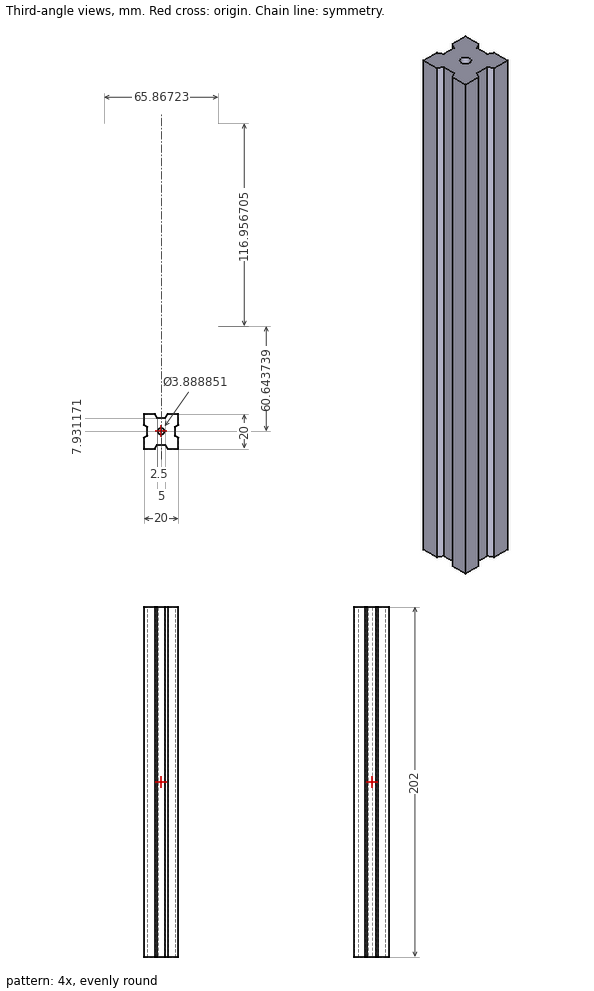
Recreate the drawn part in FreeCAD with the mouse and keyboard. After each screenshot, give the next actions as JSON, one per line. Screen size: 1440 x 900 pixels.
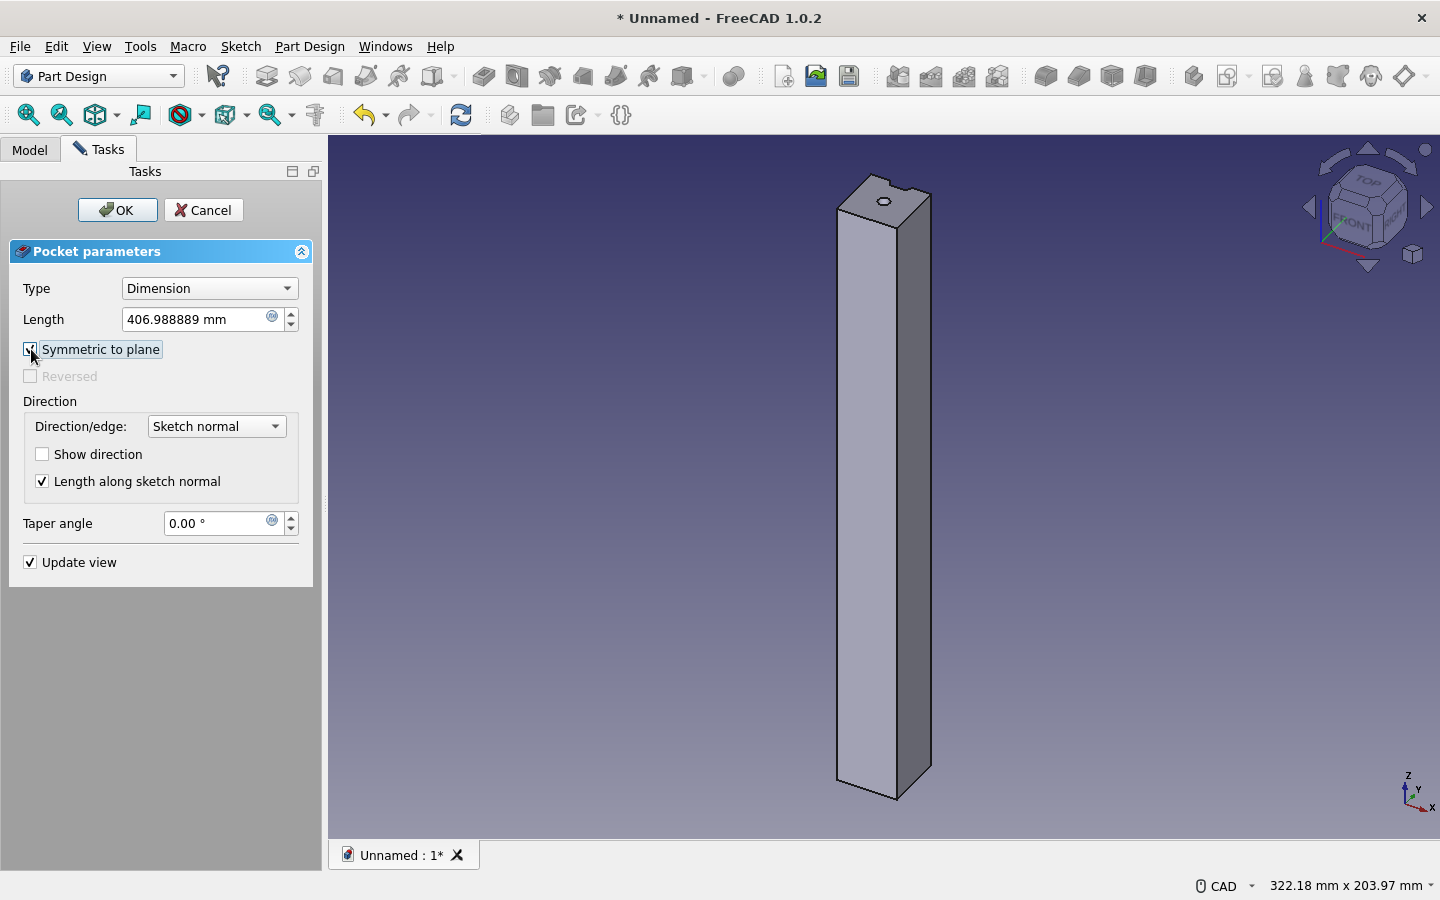
{"action": "left_click", "coordinate": [118, 210]}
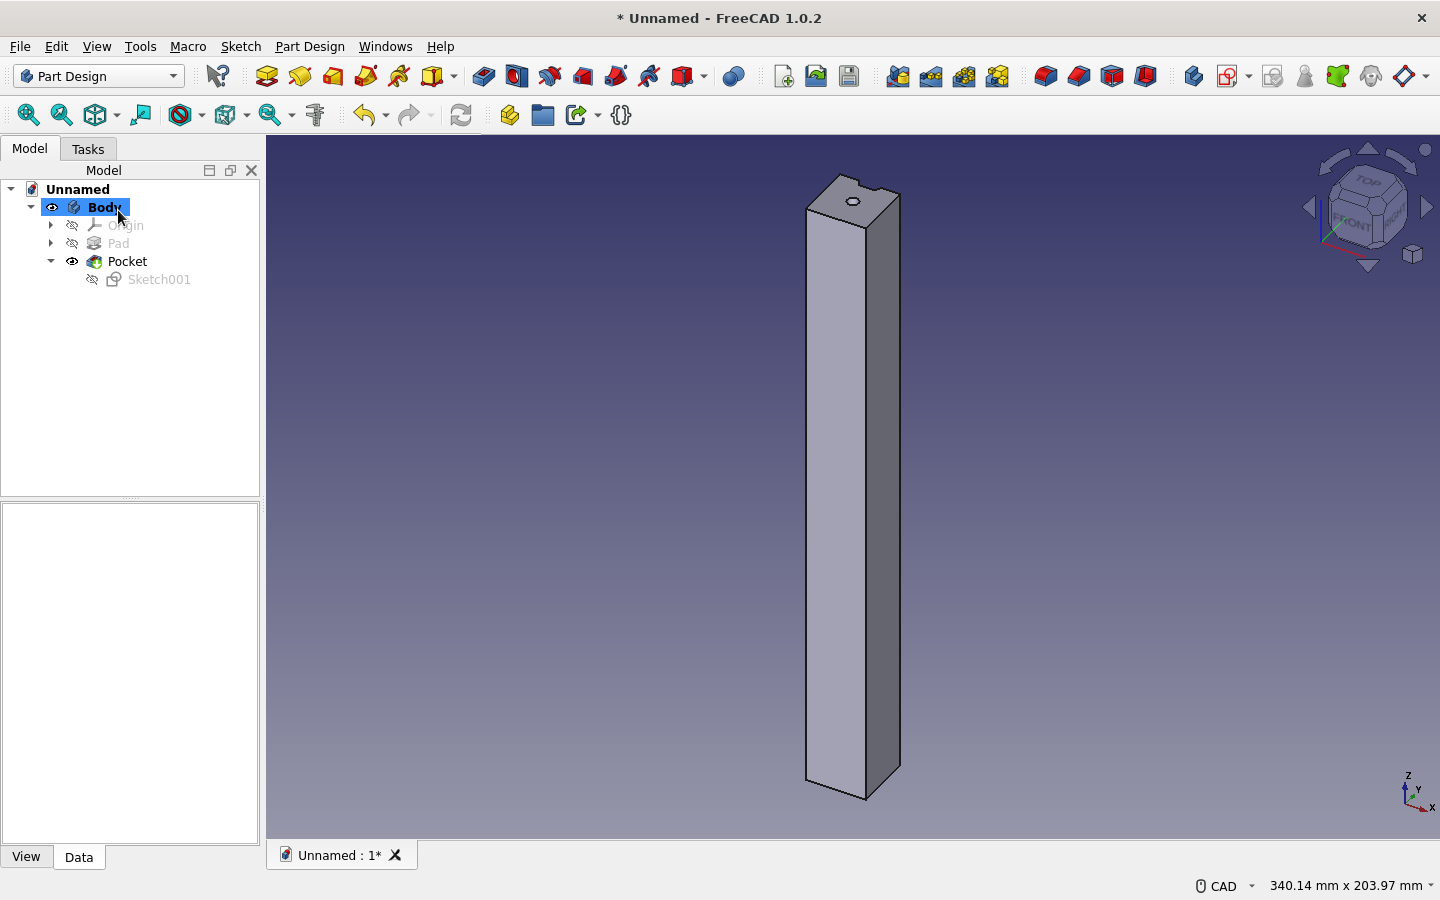
{"action": "left_click", "coordinate": [117, 261]}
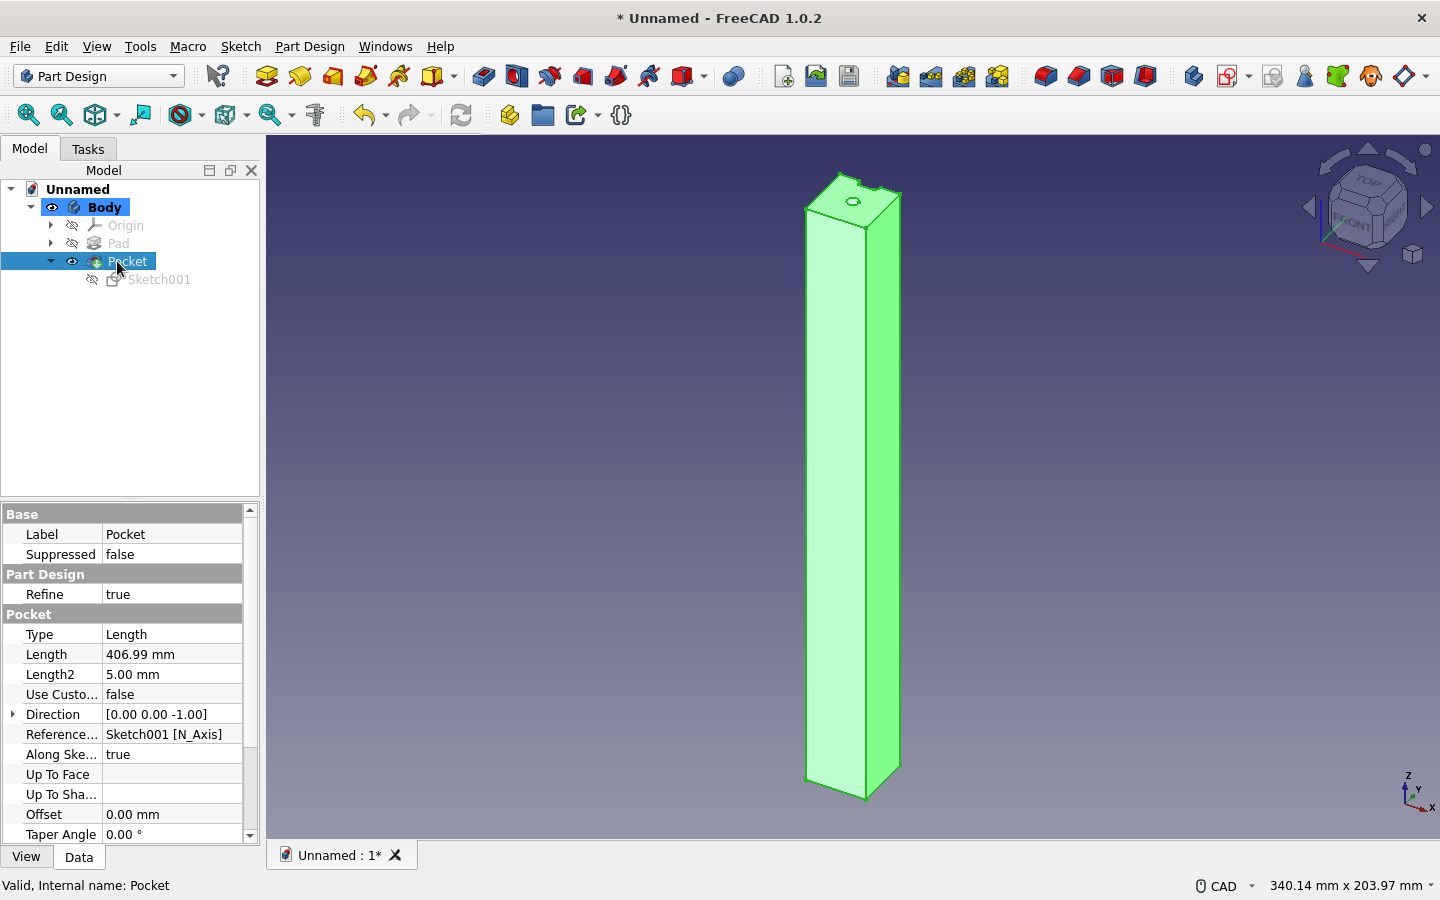
{"action": "left_click", "coordinate": [964, 76]}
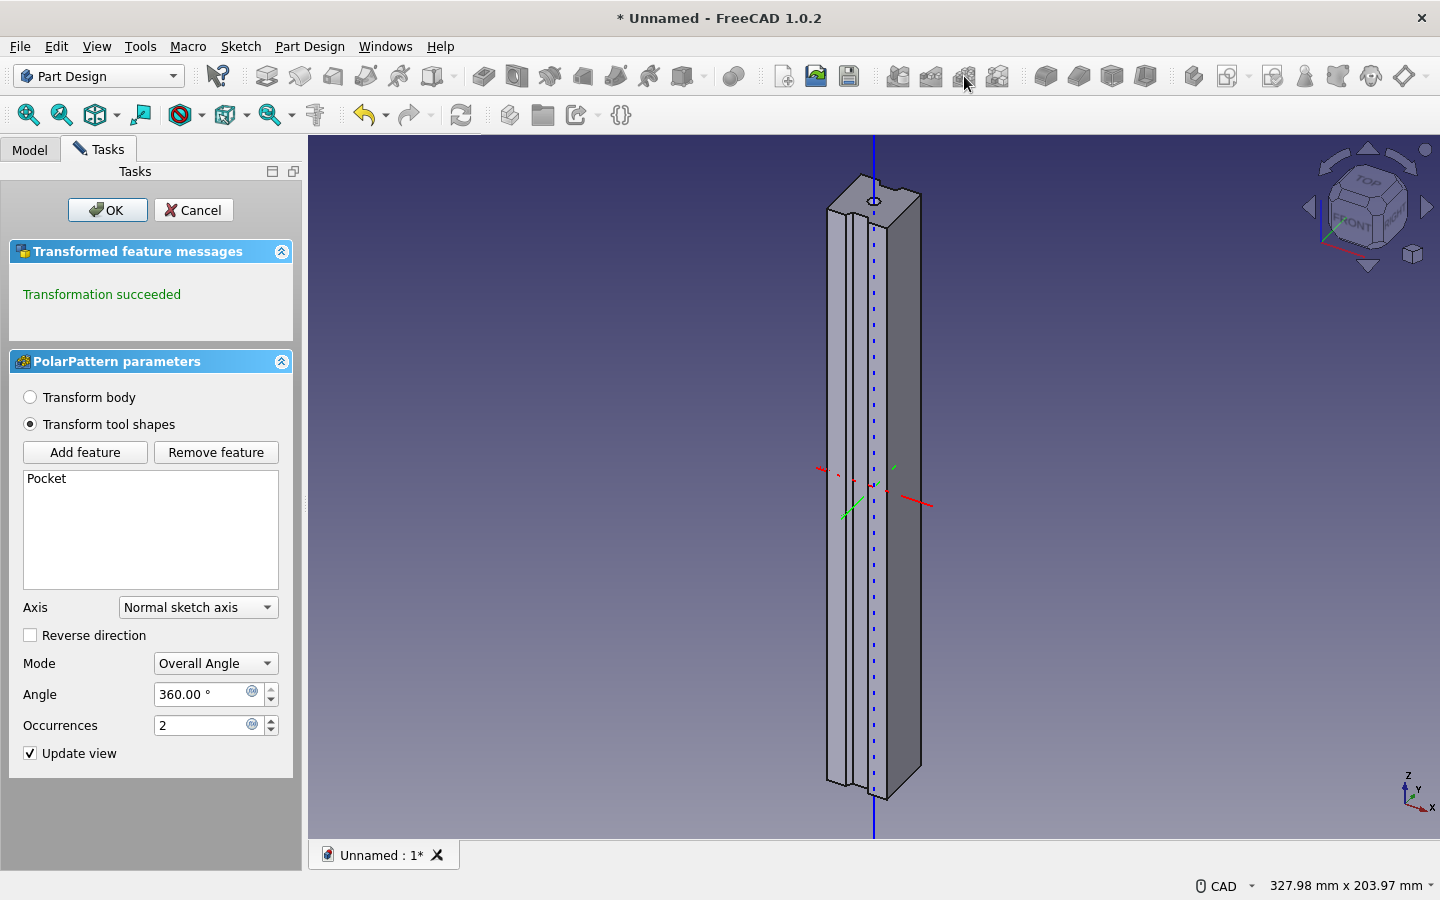
{"action": "left_click", "coordinate": [199, 608]}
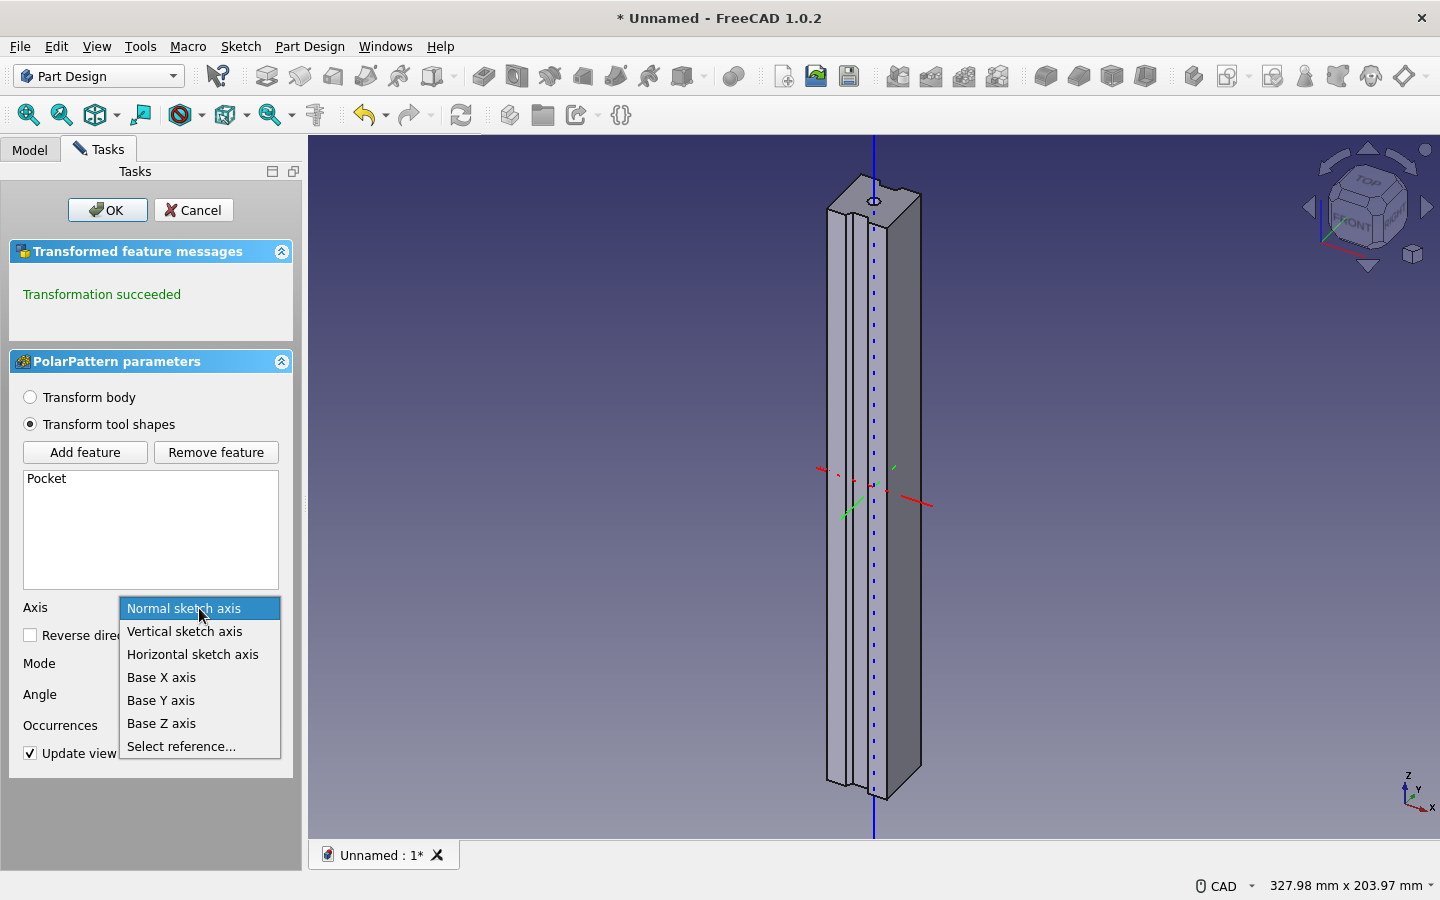
{"action": "left_click", "coordinate": [198, 724]}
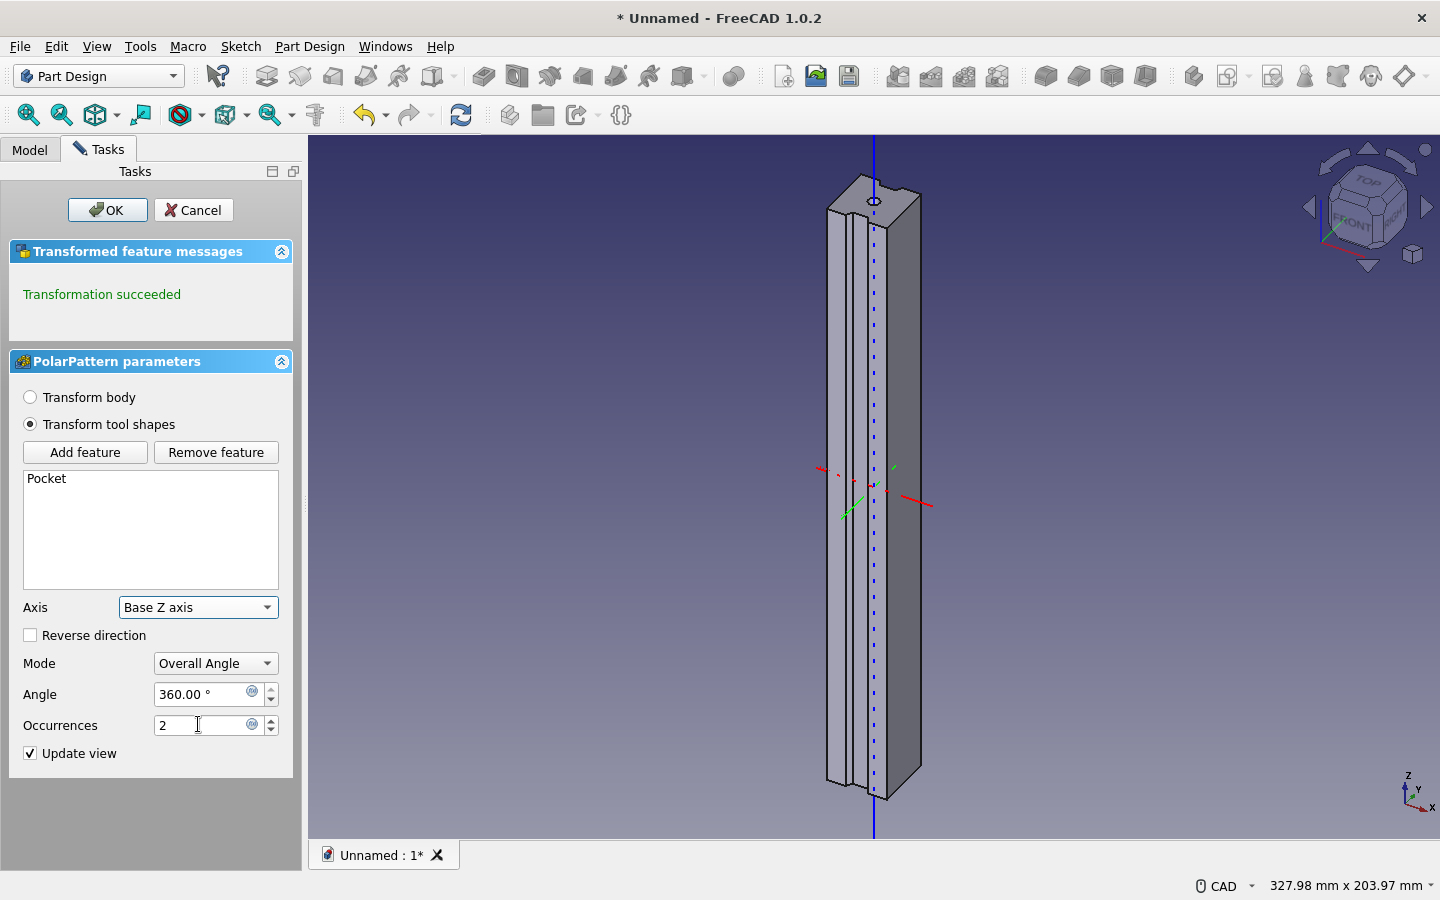
{"action": "triple_click", "coordinate": [210, 726]}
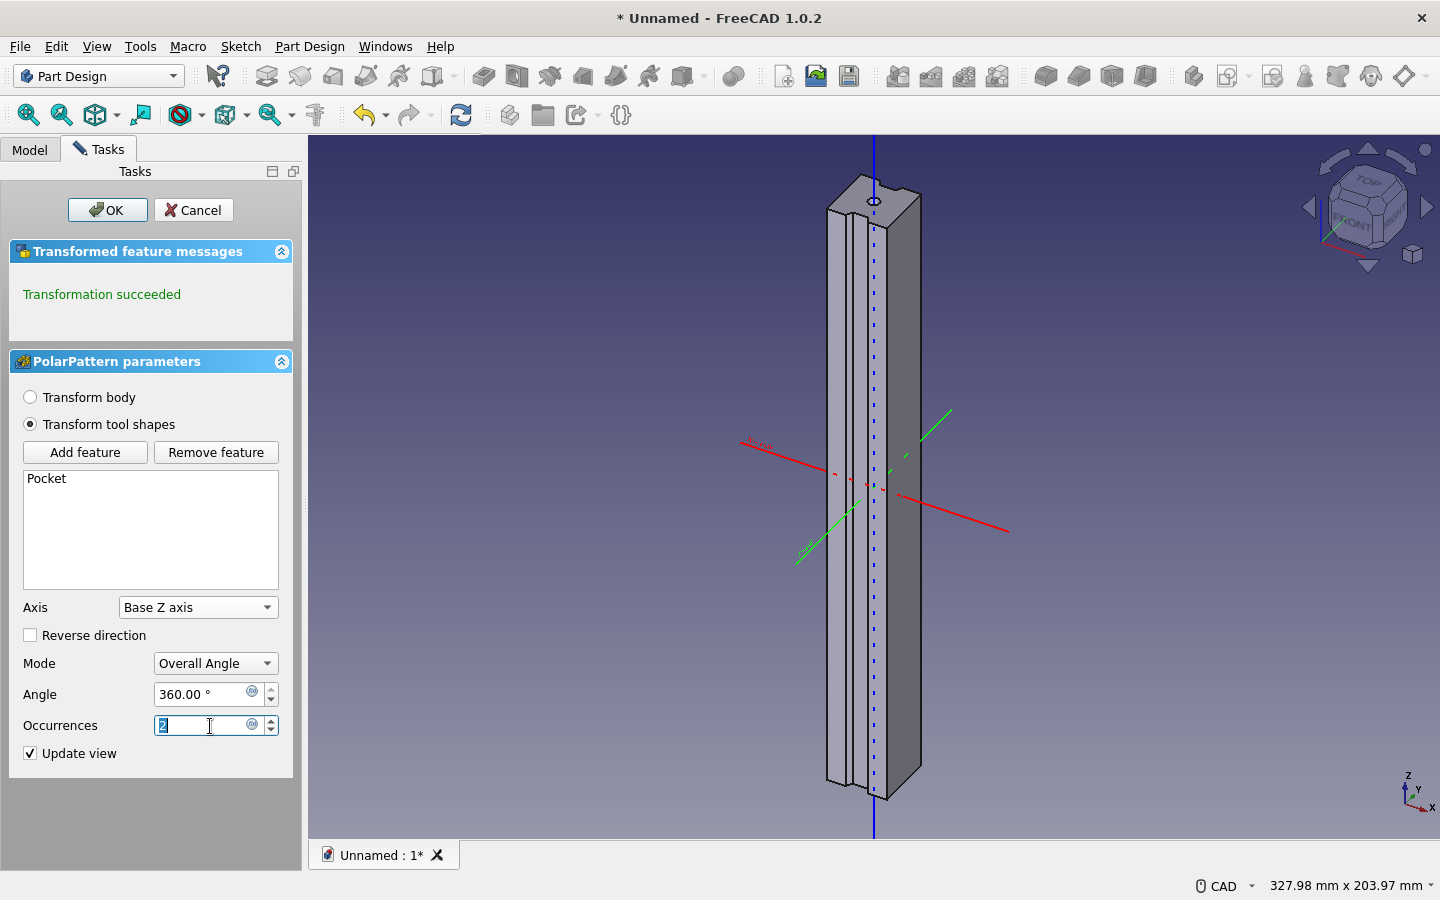
{"action": "type", "text": "4"}
{"action": "key", "text": "Tab"}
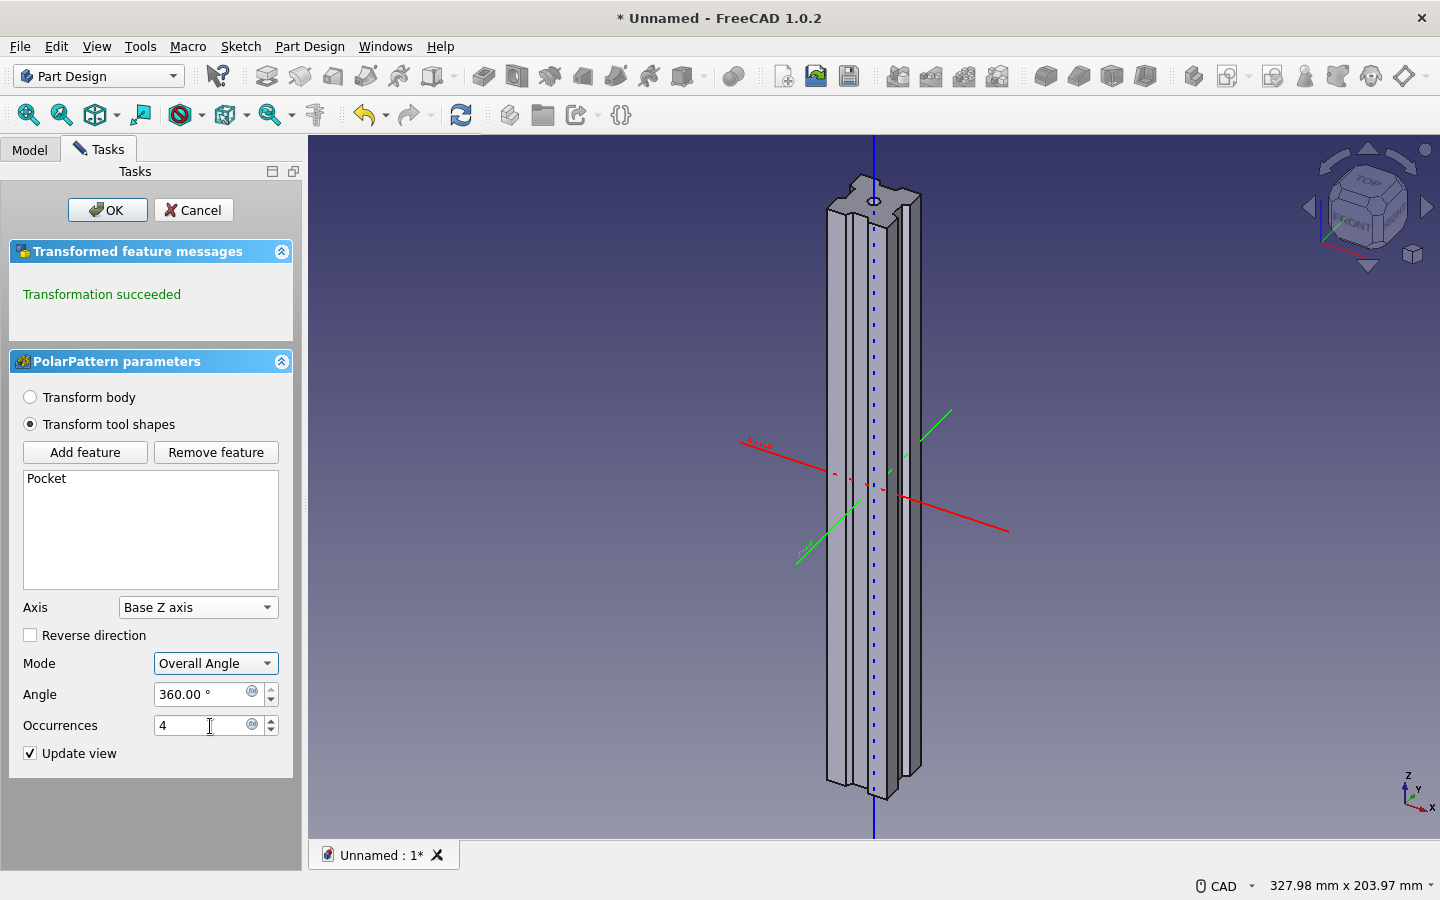
{"action": "left_click", "coordinate": [108, 210]}